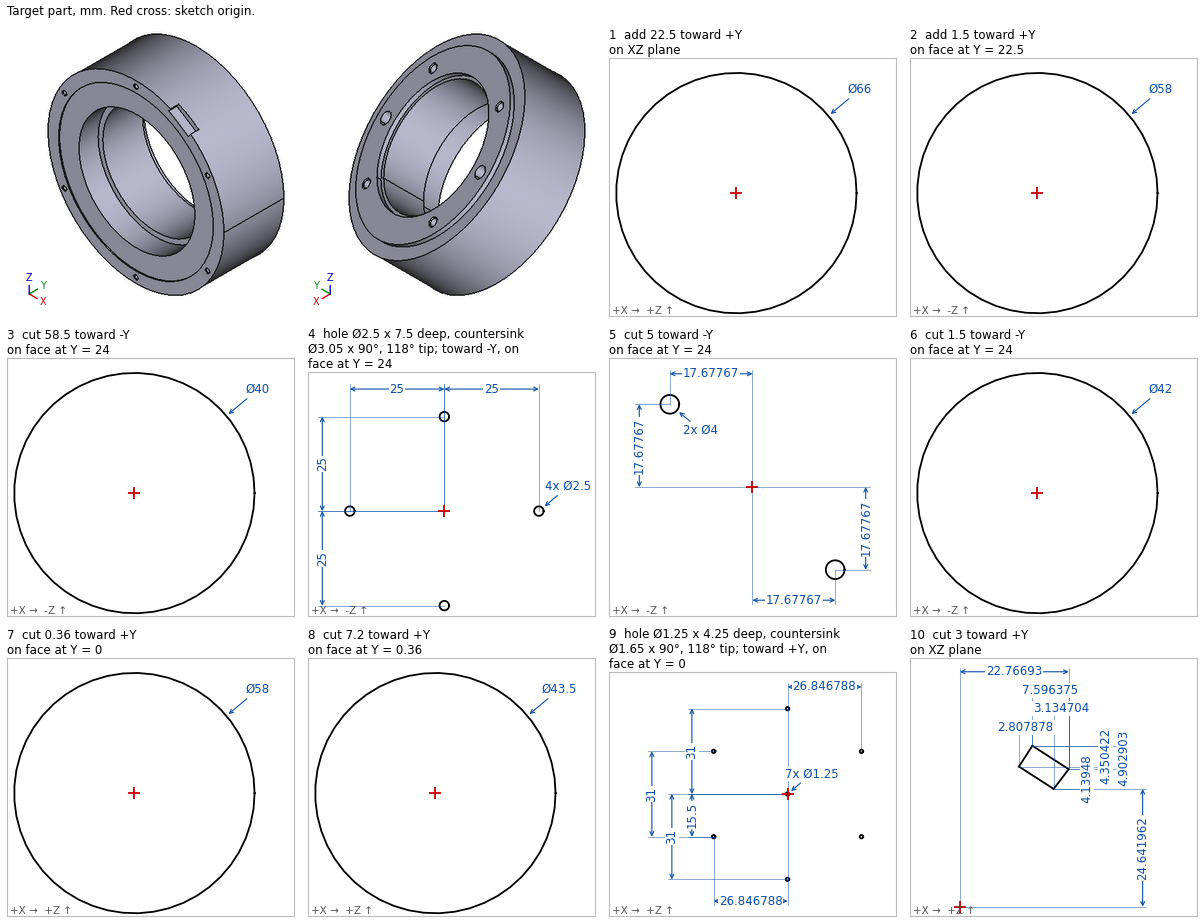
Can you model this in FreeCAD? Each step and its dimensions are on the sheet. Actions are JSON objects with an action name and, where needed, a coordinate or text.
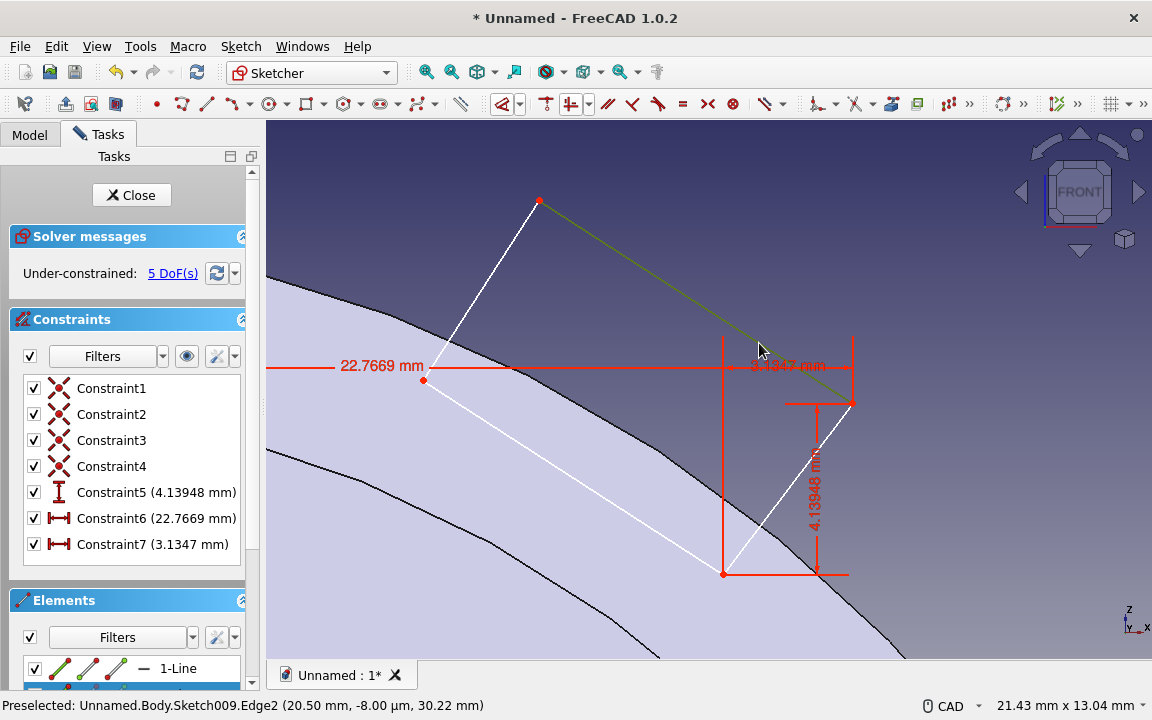
{"action": "key", "text": "l"}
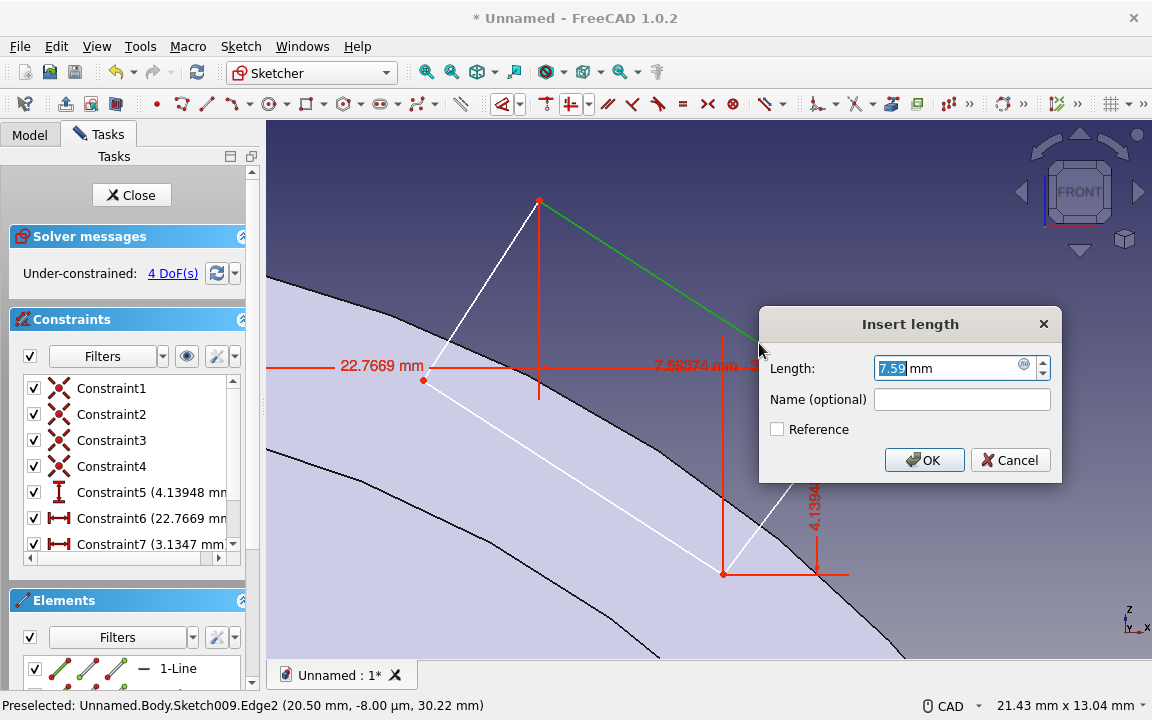
{"action": "type", "text": "7.596375"}
{"action": "key", "text": "Return"}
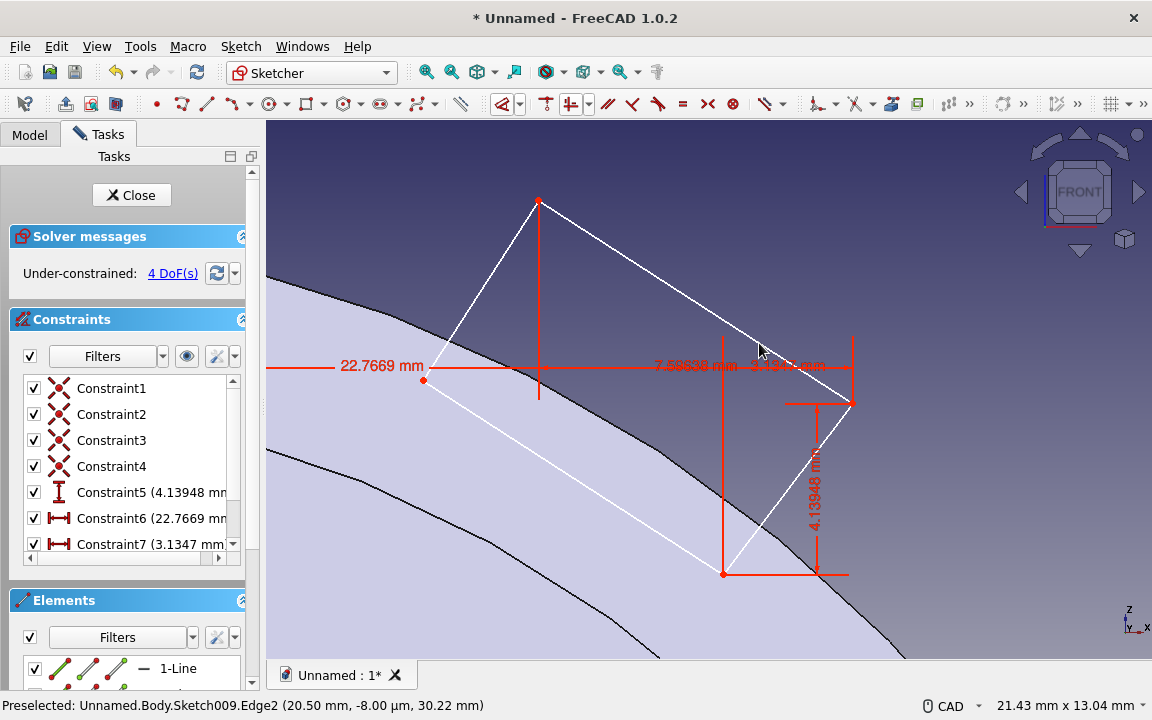
{"action": "left_click", "coordinate": [759, 343]}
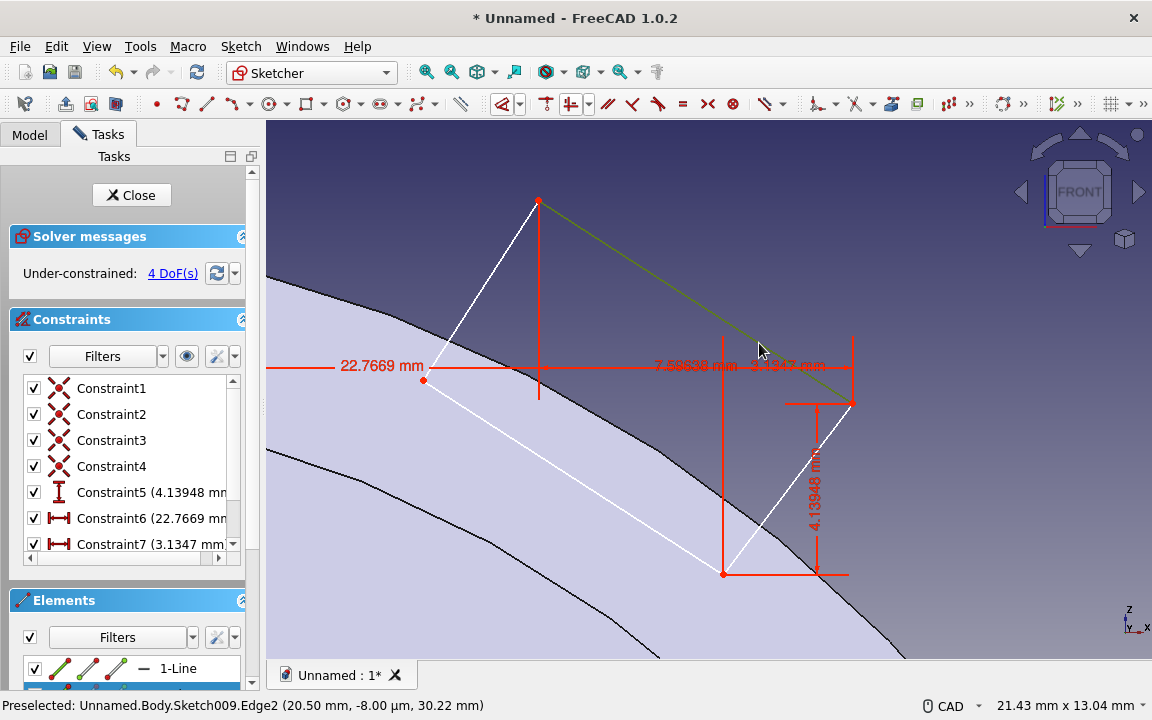
{"action": "left_click", "coordinate": [520, 104]}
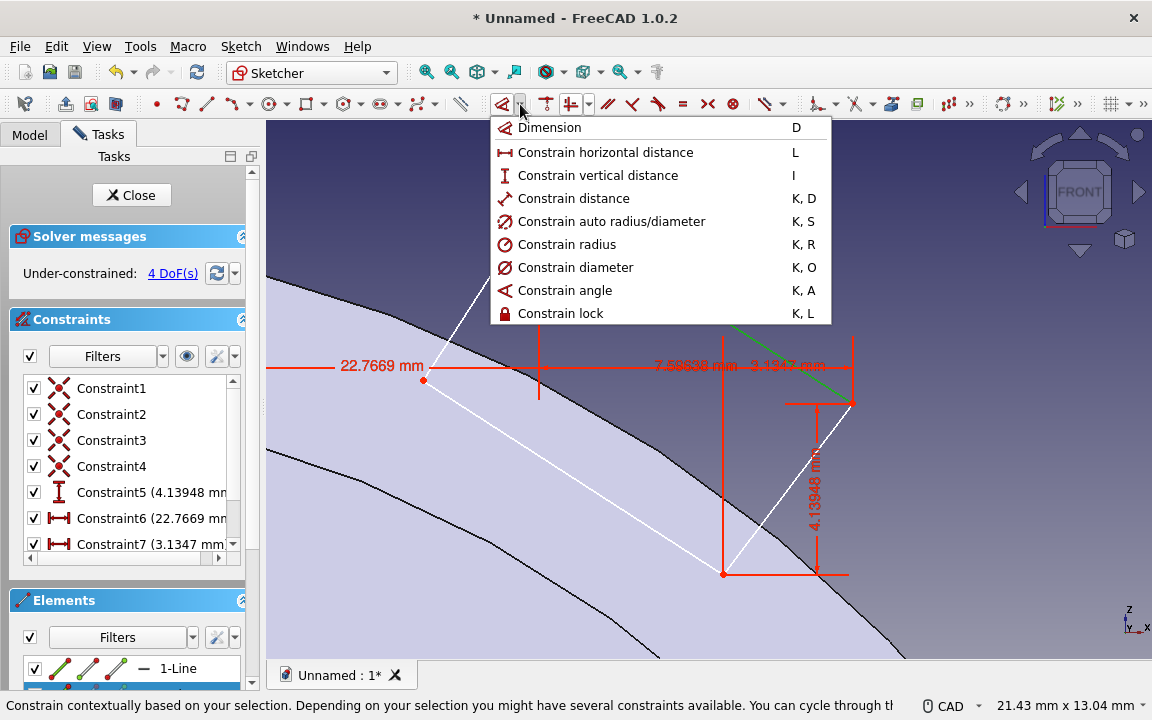
{"action": "left_click", "coordinate": [661, 176]}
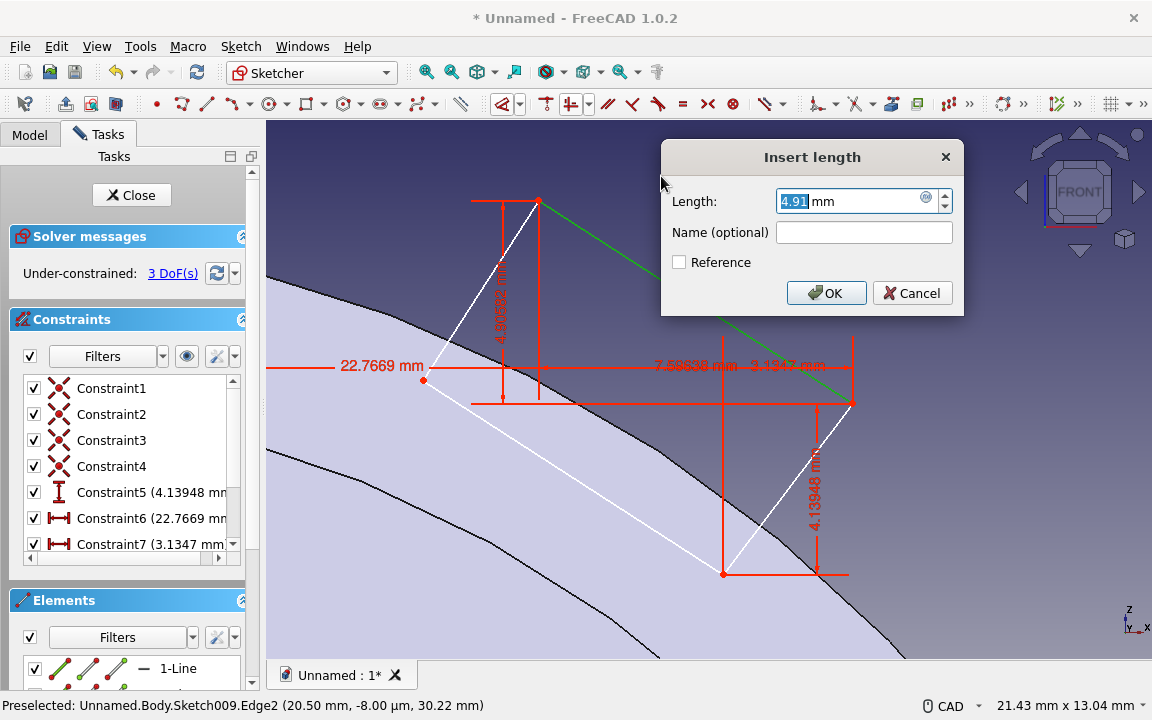
{"action": "type", "text": "4.902903"}
{"action": "key", "text": "Return"}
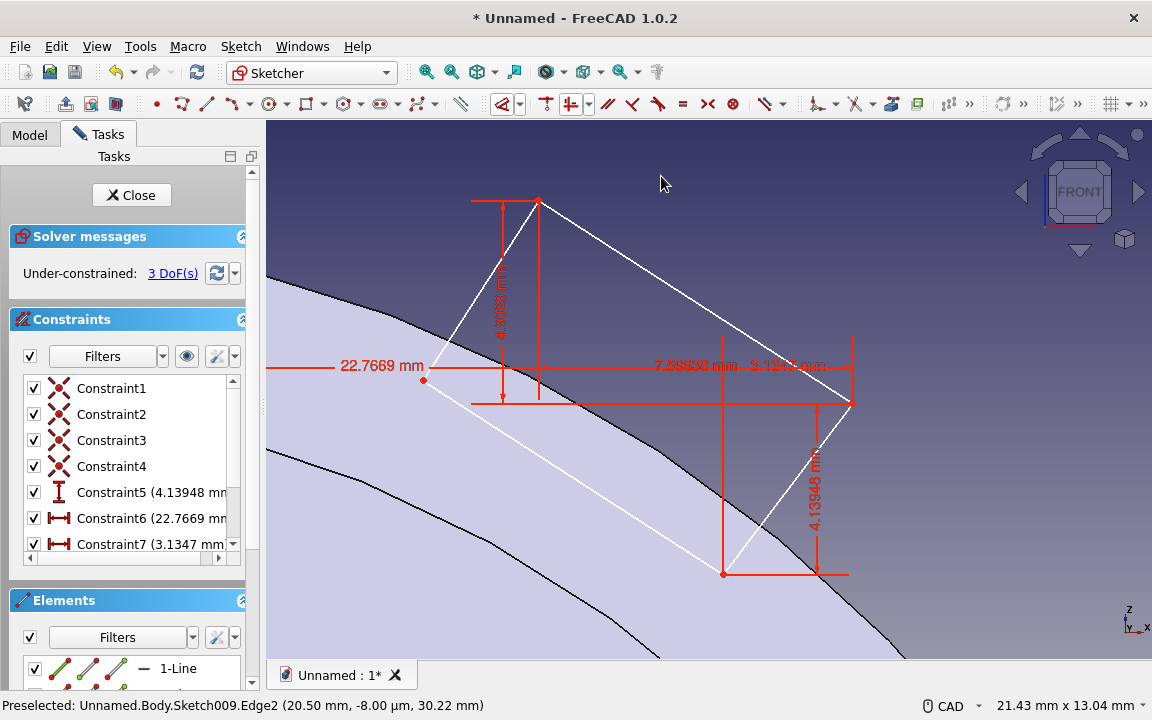
{"action": "left_click", "coordinate": [504, 255]}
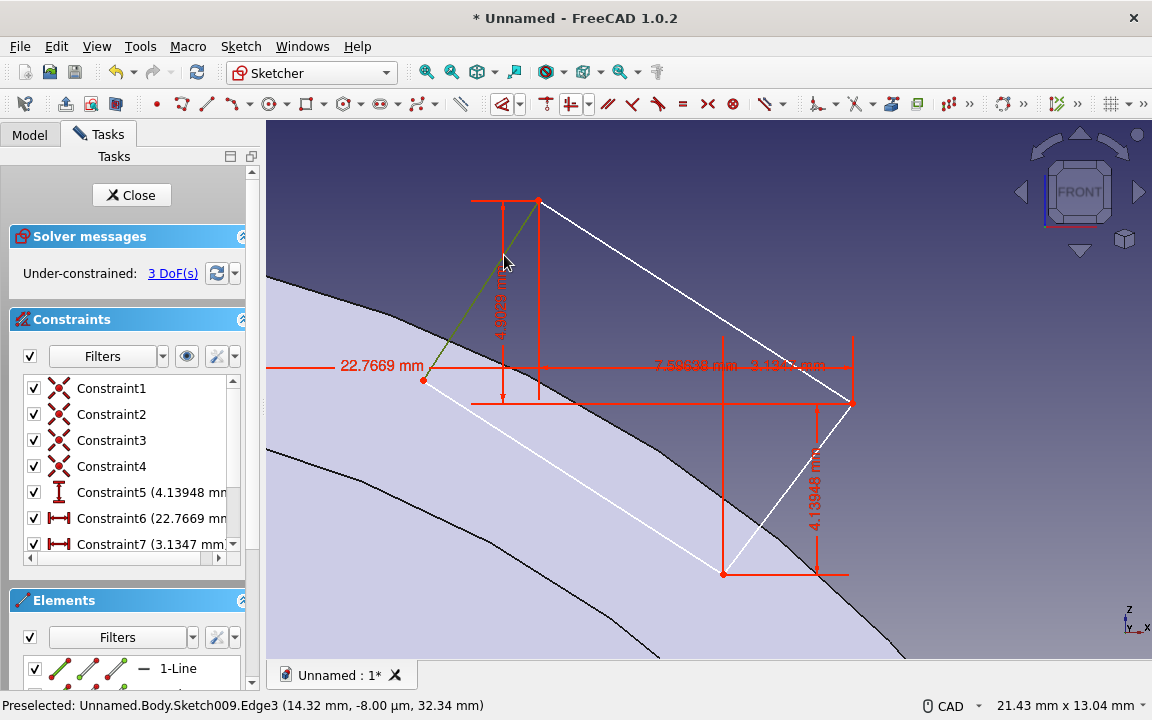
{"action": "key", "text": "l"}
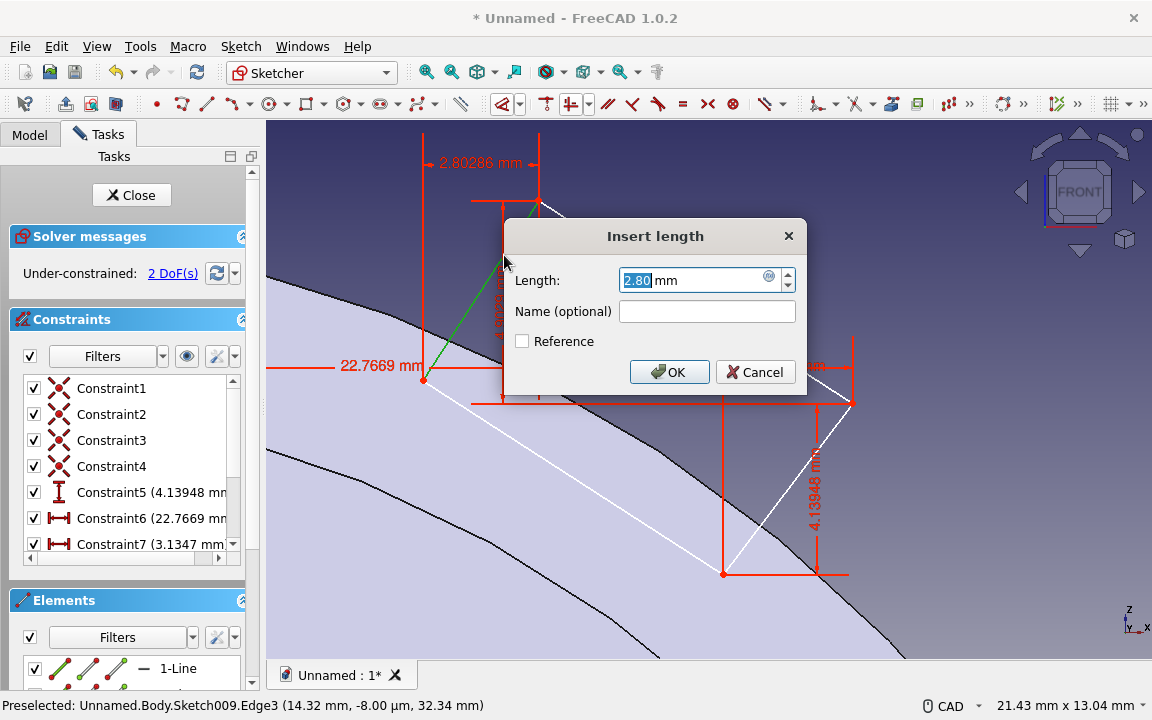
{"action": "type", "text": "2.807878"}
{"action": "key", "text": "Return"}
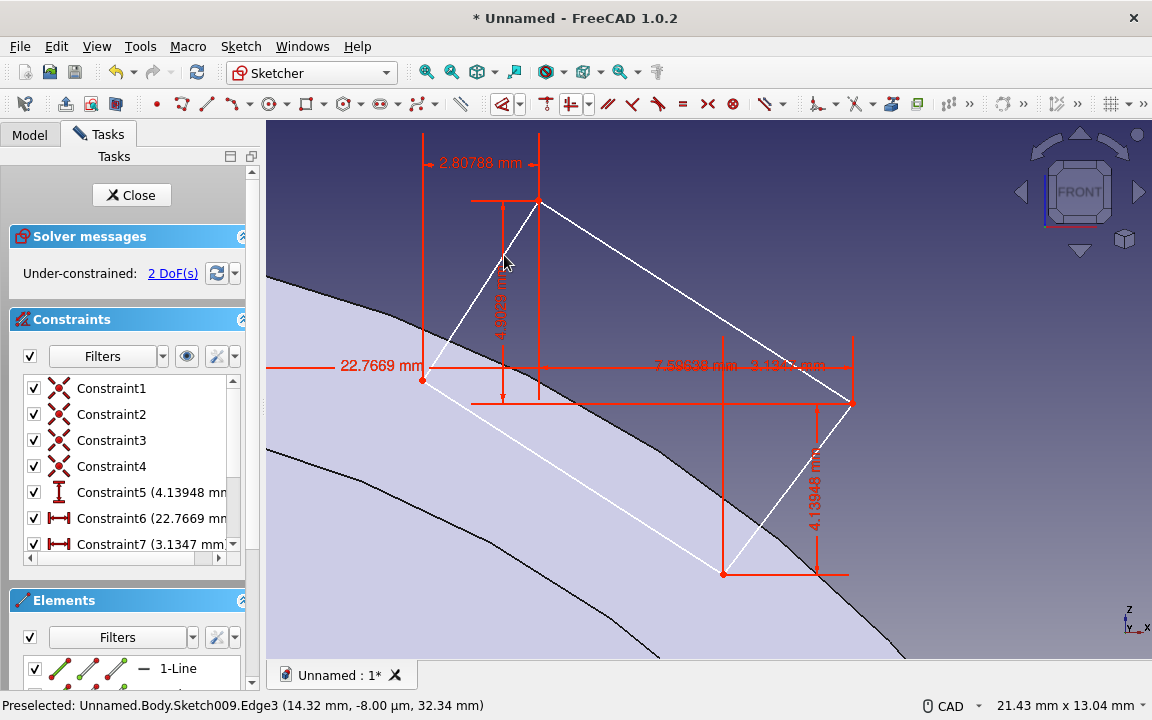
{"action": "left_click", "coordinate": [504, 255]}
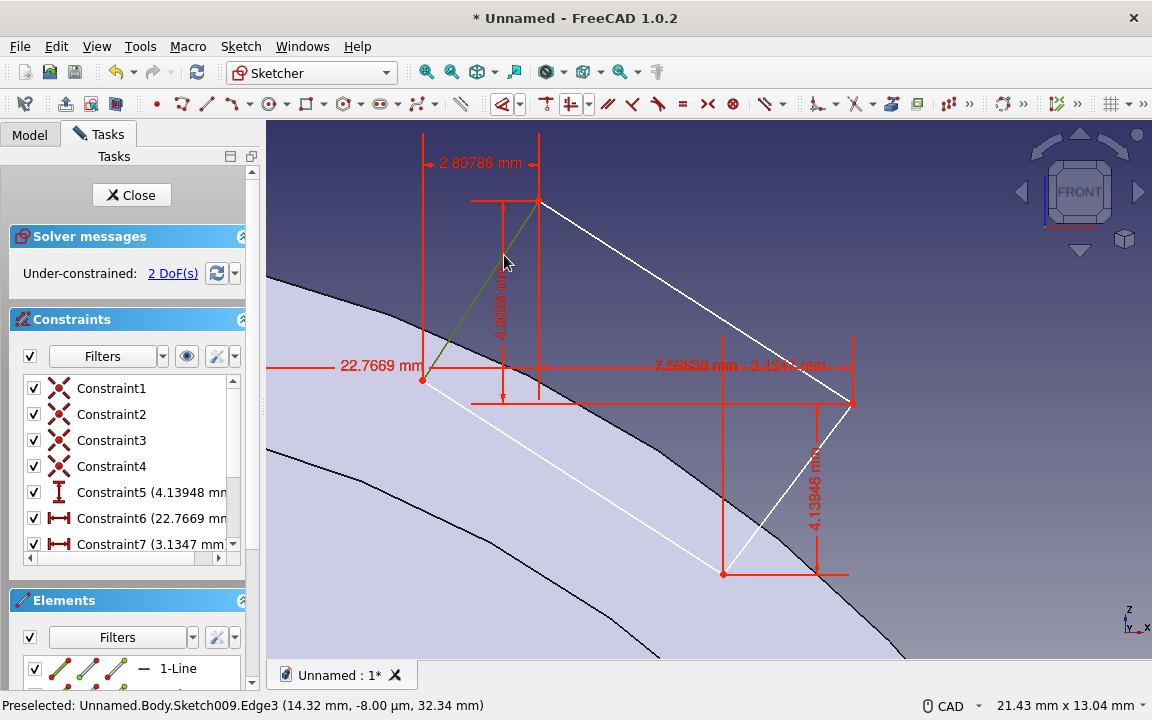
{"action": "key", "text": "i"}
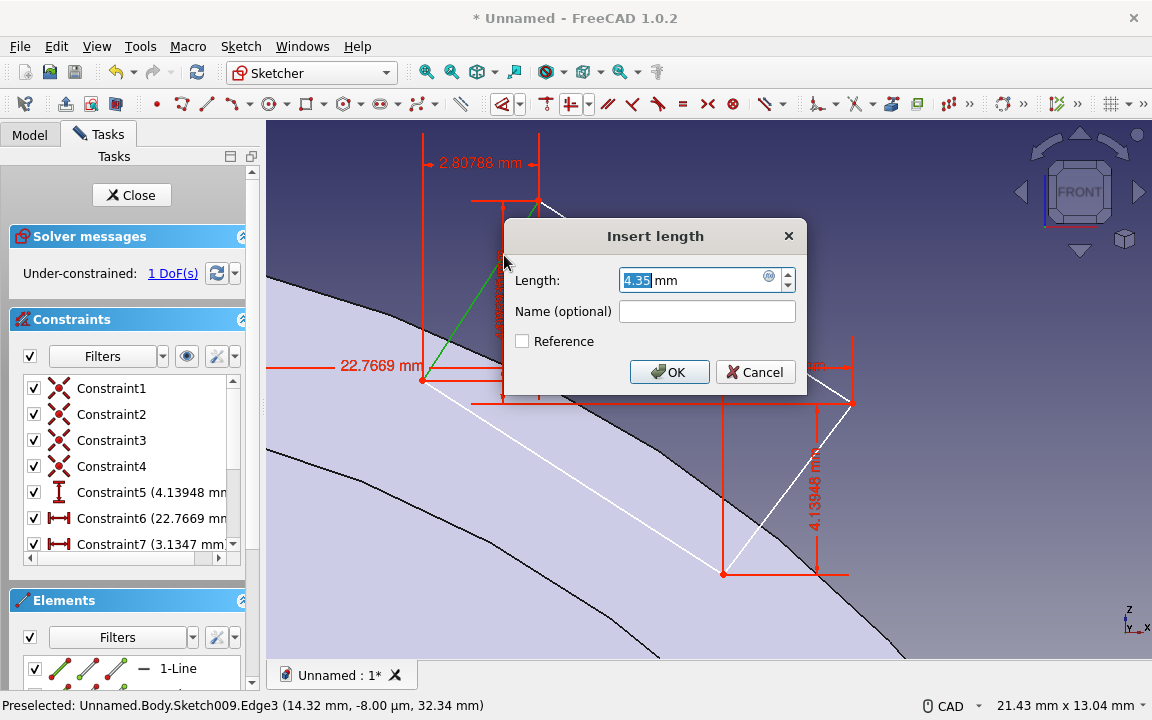
{"action": "type", "text": "4.350422"}
{"action": "key", "text": "Return"}